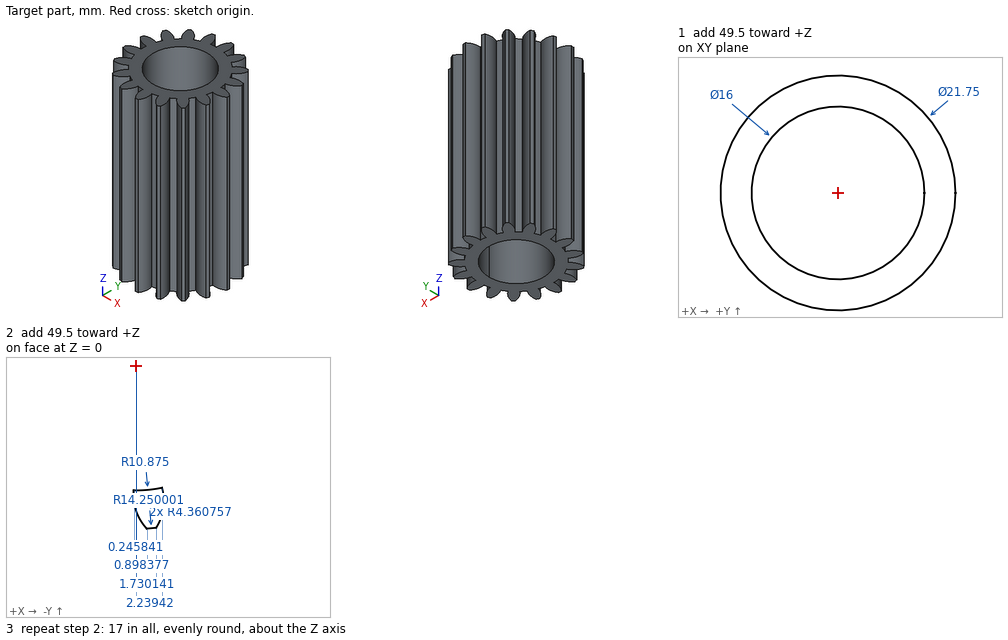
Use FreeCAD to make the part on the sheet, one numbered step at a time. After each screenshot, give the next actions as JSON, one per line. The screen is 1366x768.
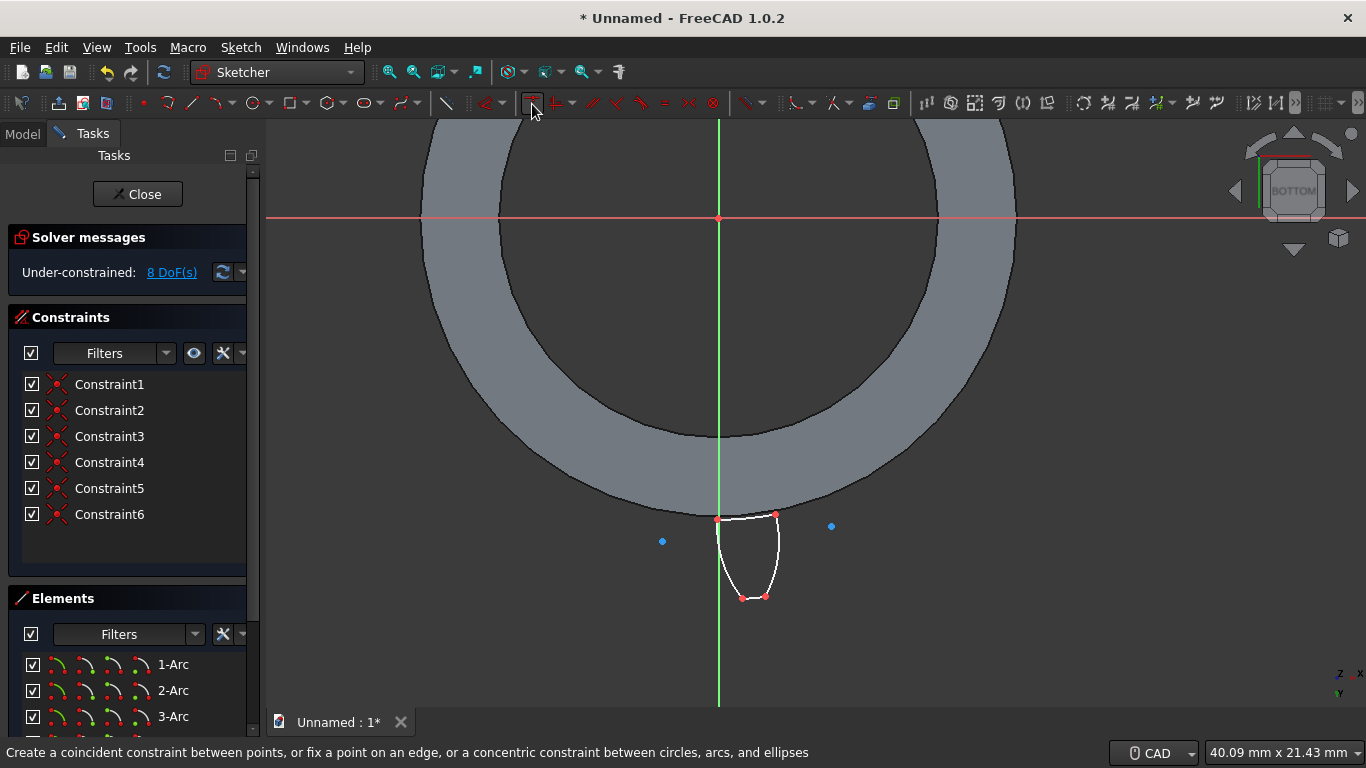
{"action": "left_click", "coordinate": [775, 573]}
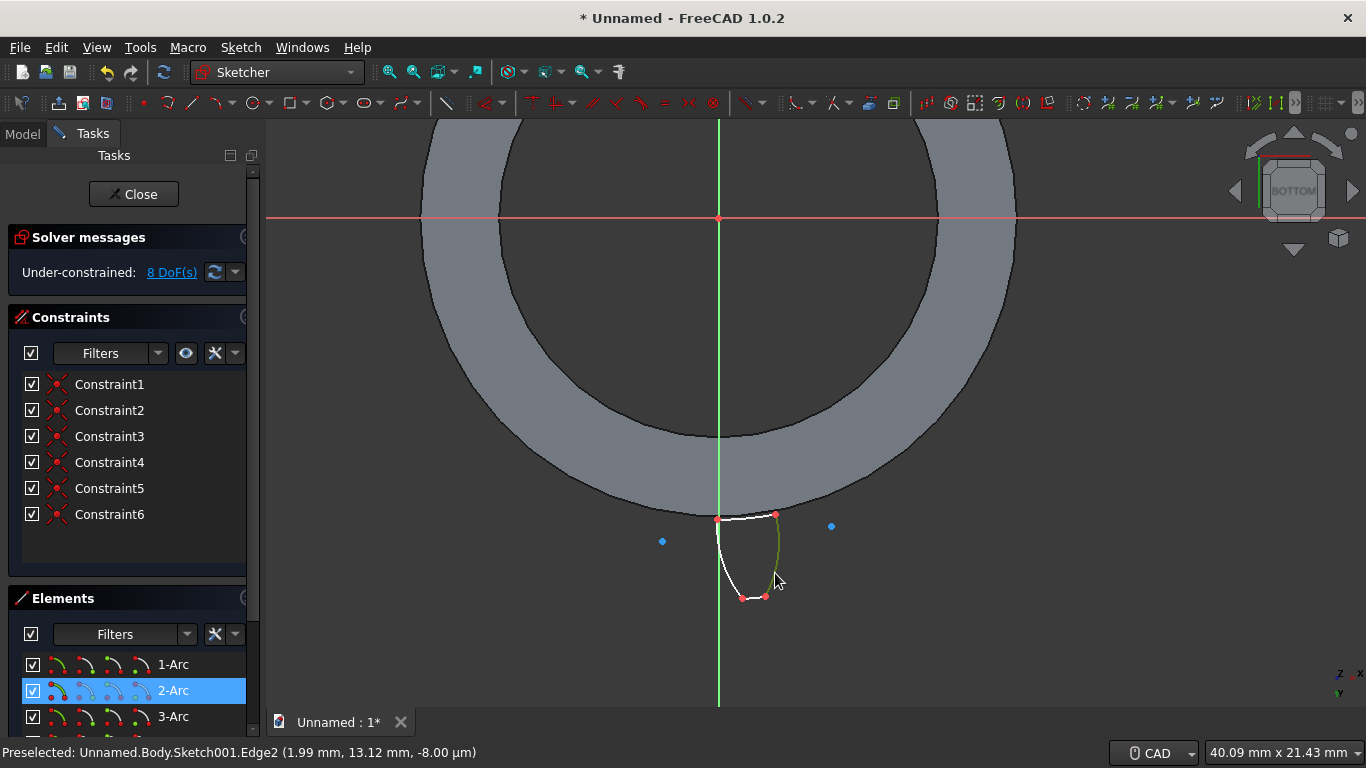
{"action": "left_click", "coordinate": [719, 545]}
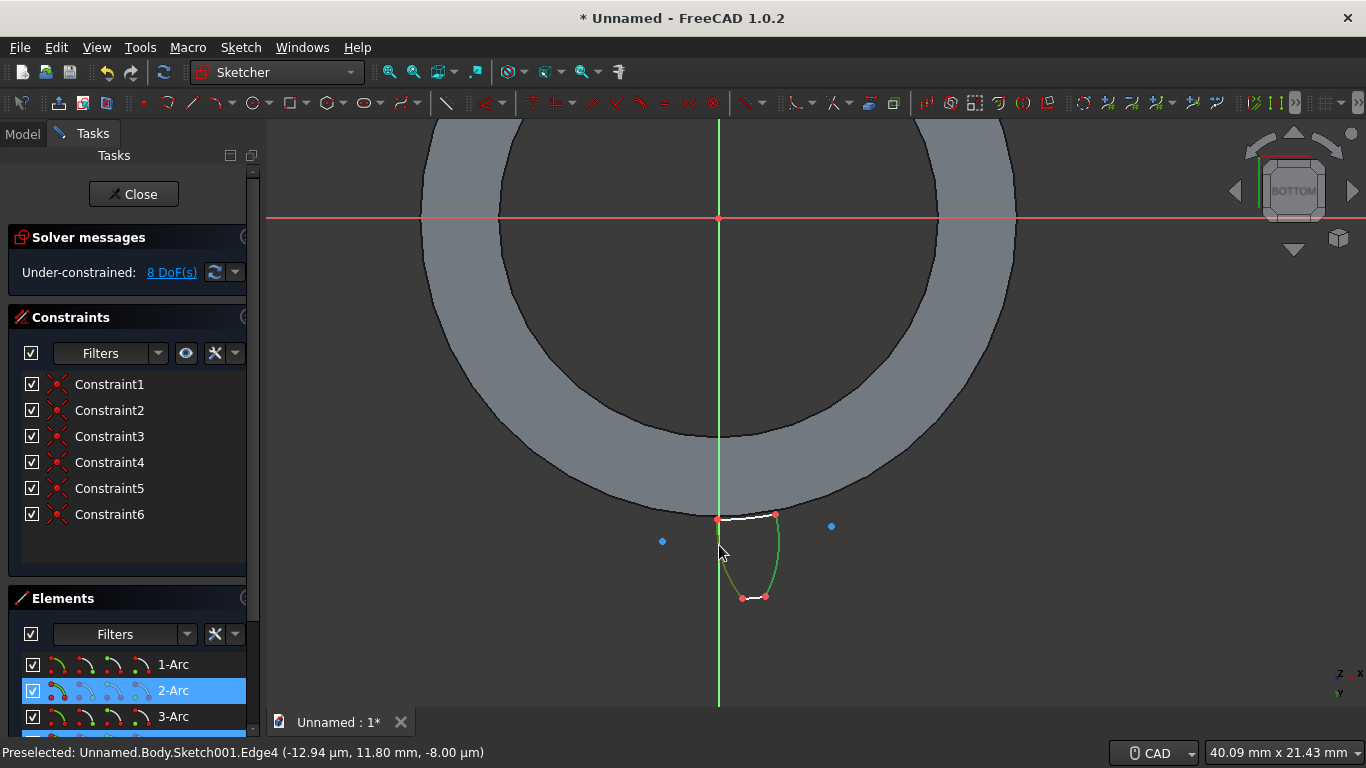
{"action": "left_click", "coordinate": [666, 104]}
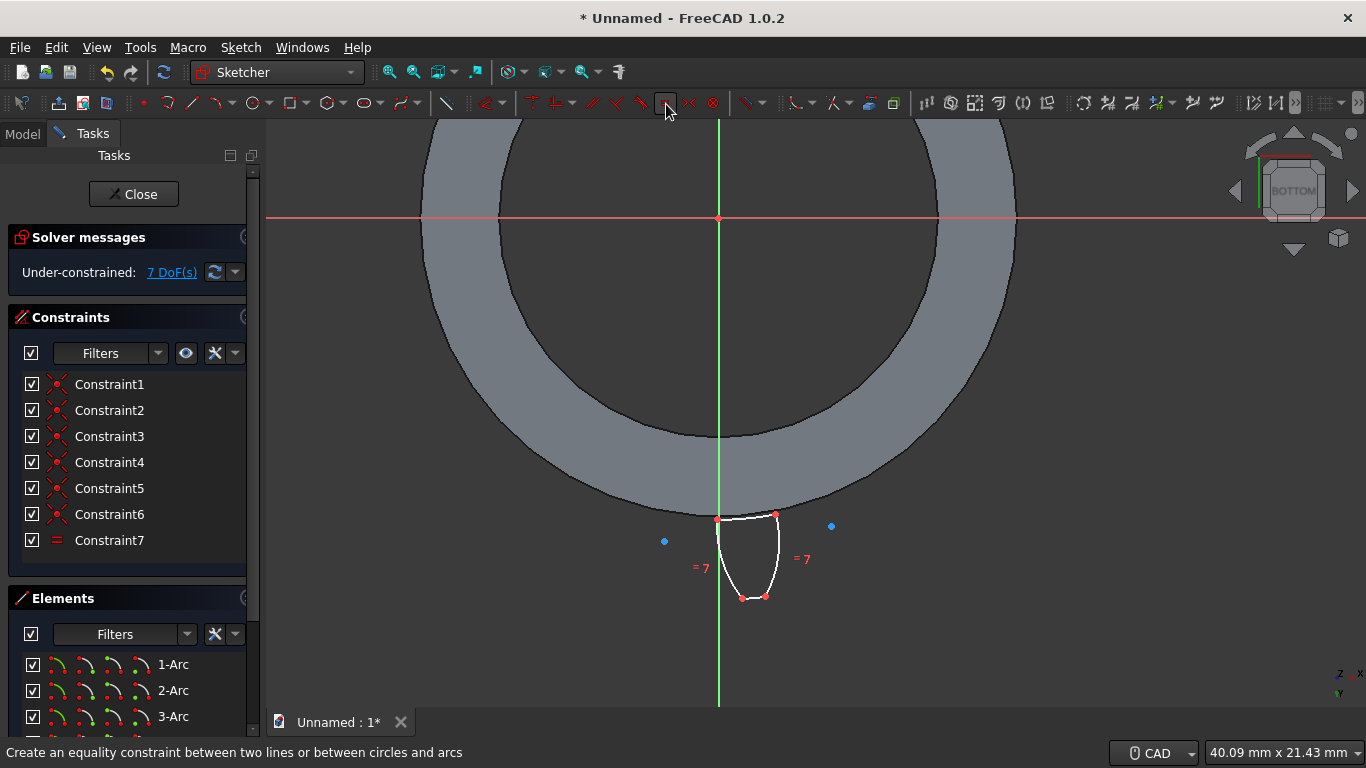
{"action": "left_click", "coordinate": [486, 104]}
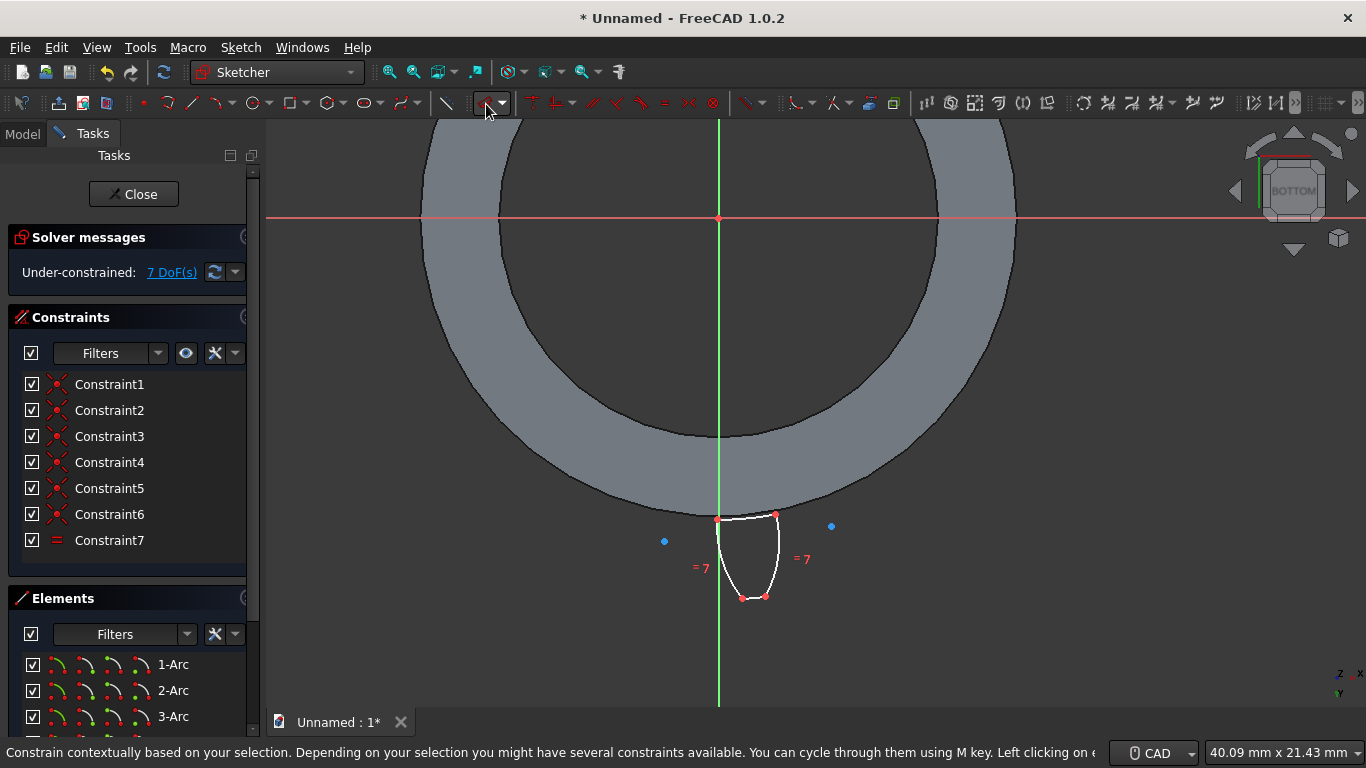
{"action": "left_click", "coordinate": [735, 519]}
{"action": "left_click", "coordinate": [737, 551]}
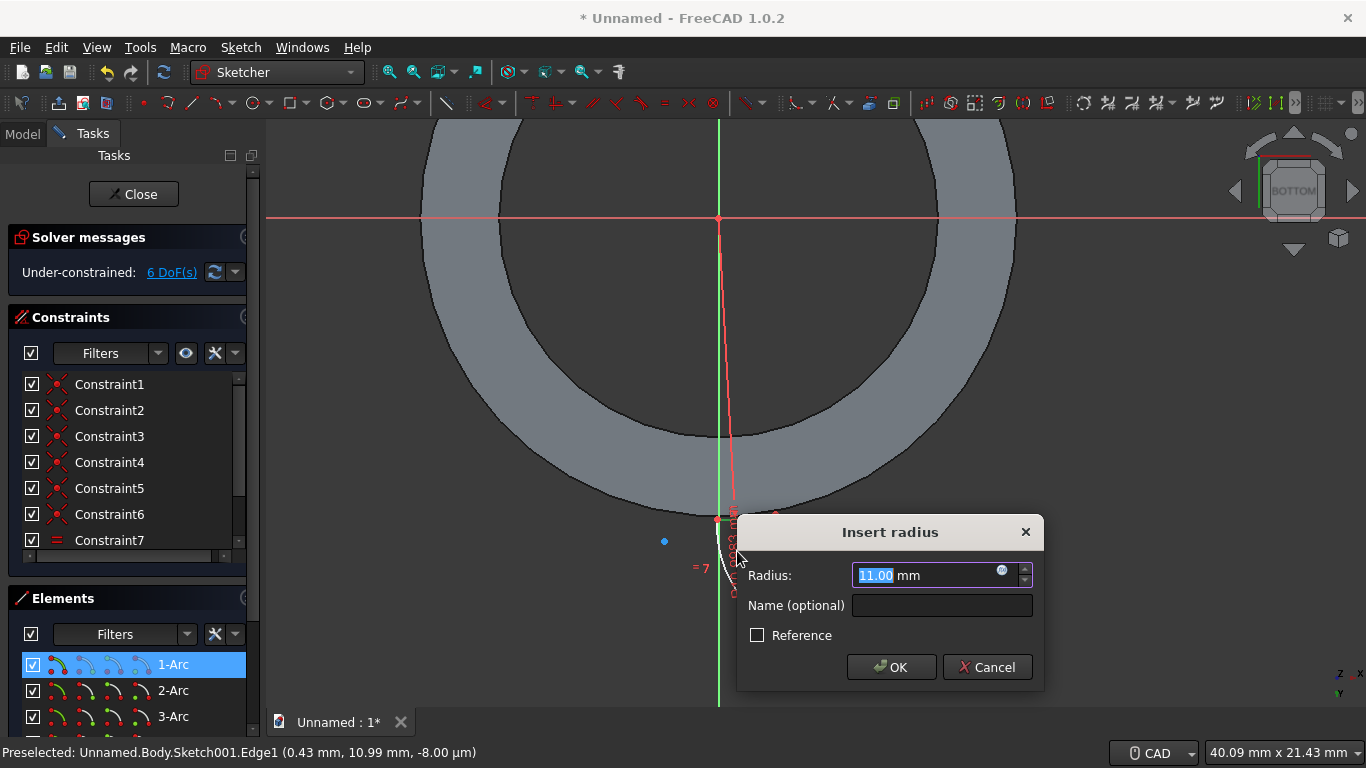
{"action": "type", "text": "10.875"}
{"action": "key", "text": "Return"}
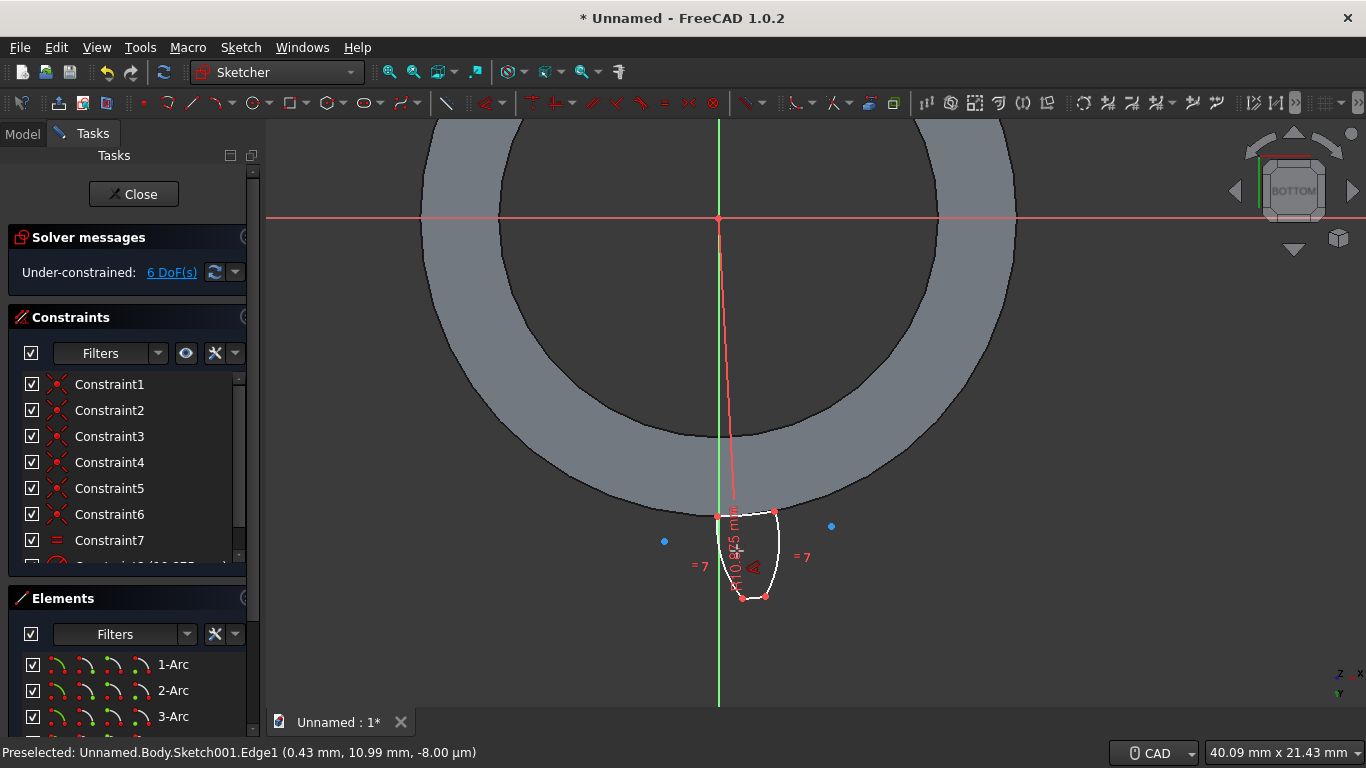
{"action": "left_click", "coordinate": [775, 572]}
{"action": "left_click", "coordinate": [806, 580]}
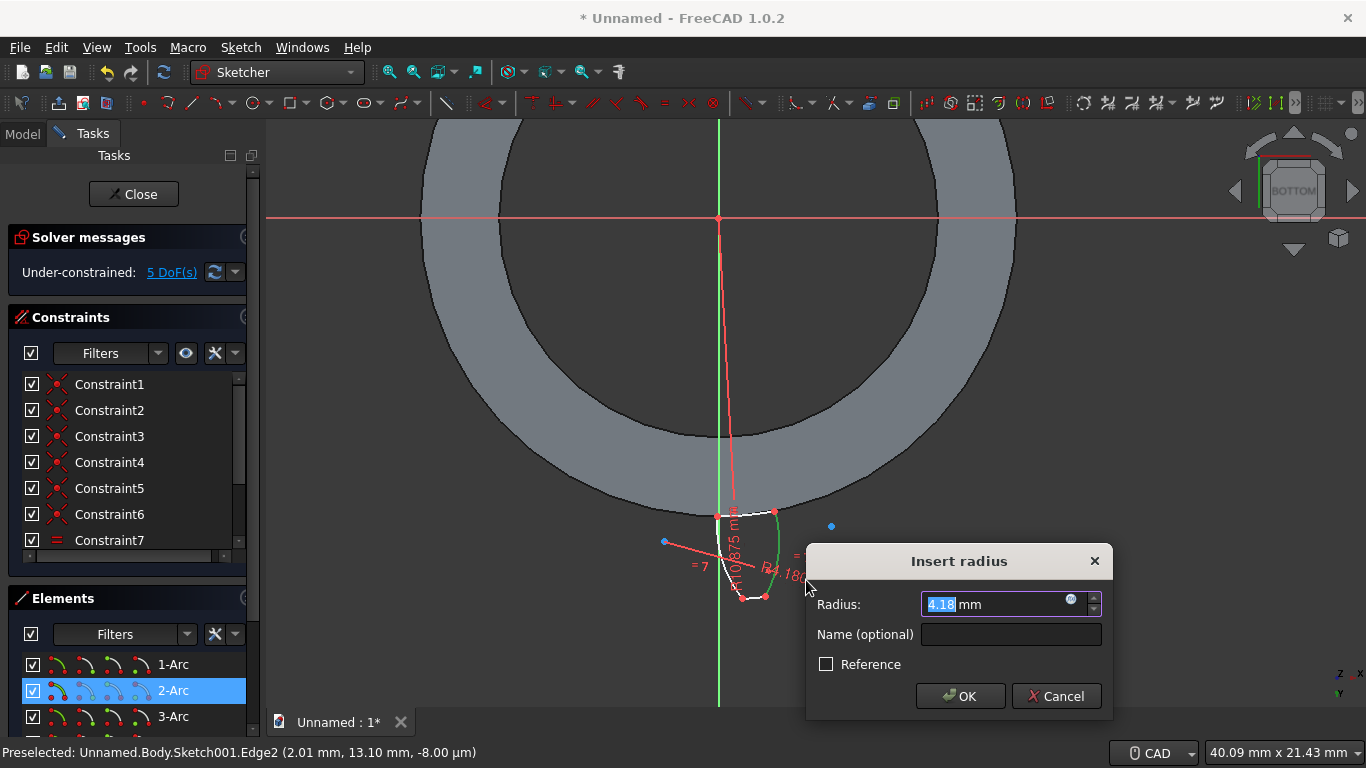
{"action": "type", "text": "4.360757"}
{"action": "key", "text": "Return"}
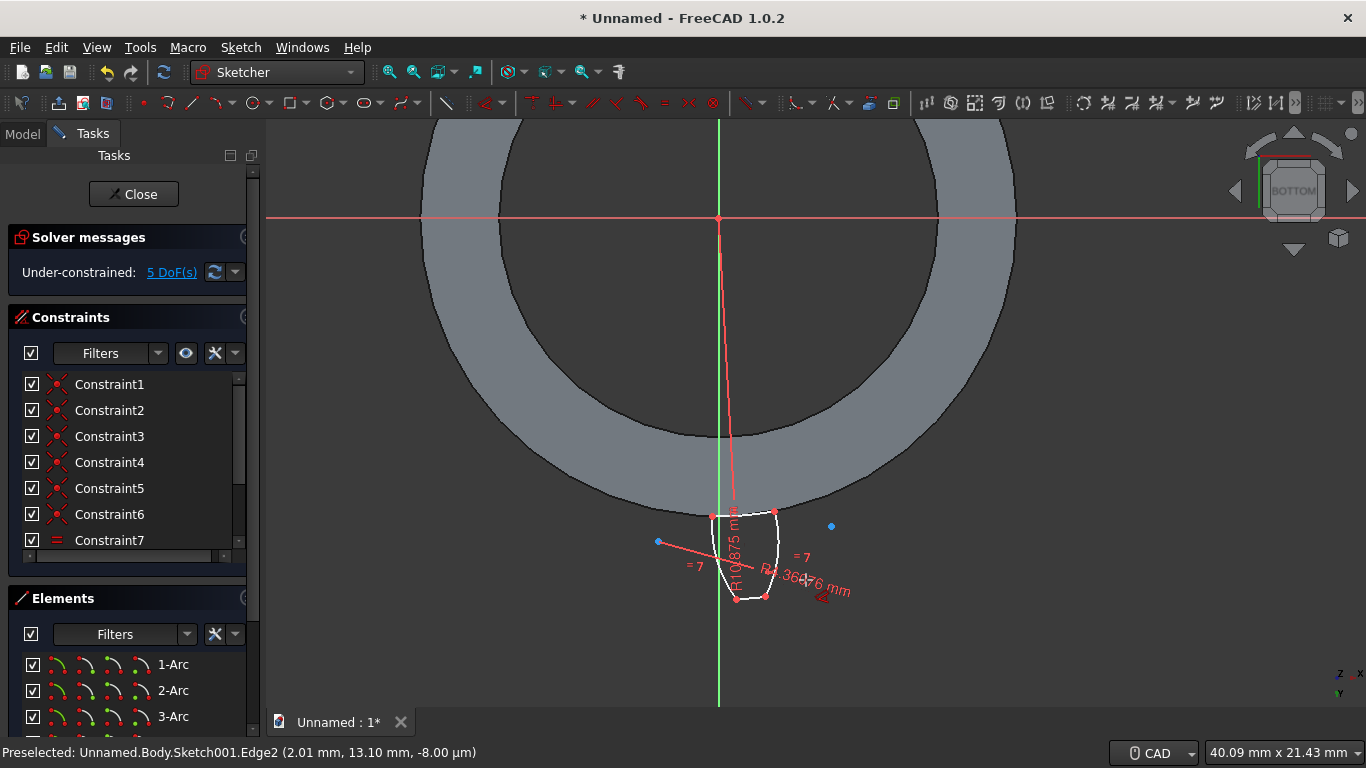
{"action": "left_click", "coordinate": [751, 598]}
{"action": "left_click", "coordinate": [754, 630]}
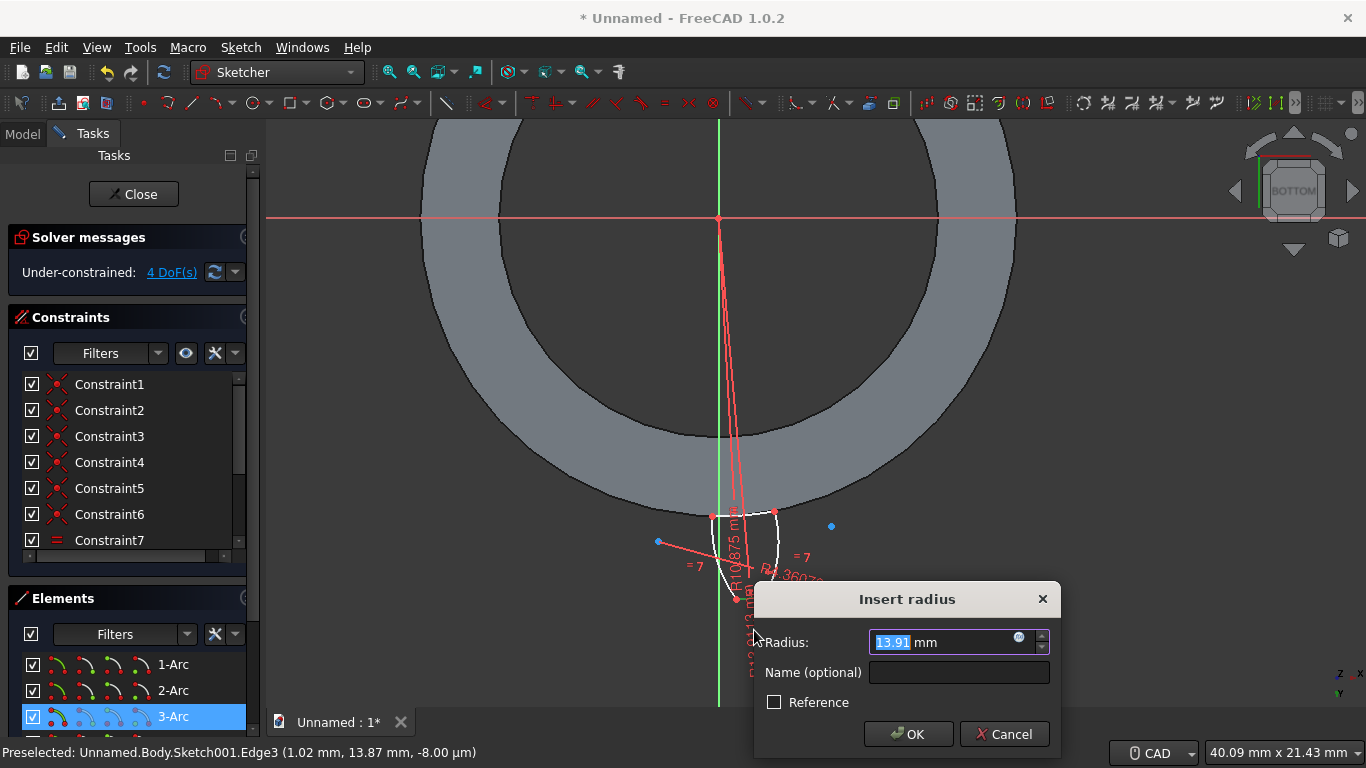
{"action": "type", "text": "14.250001"}
{"action": "key", "text": "Return"}